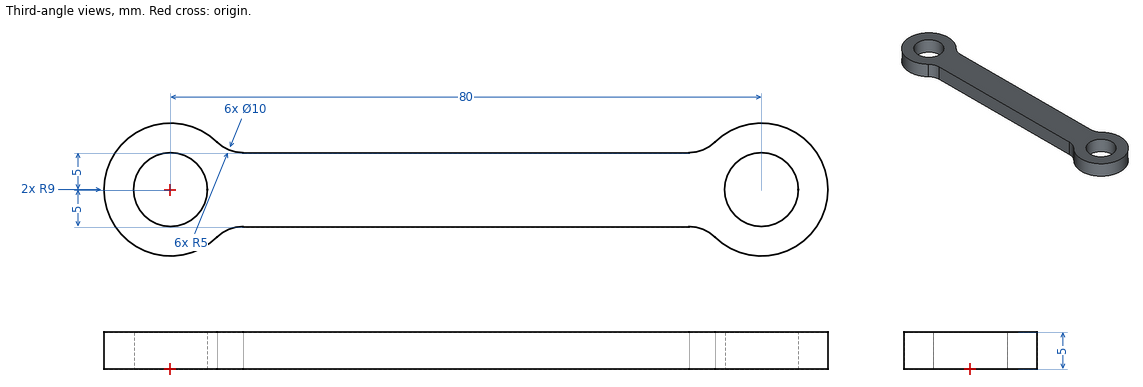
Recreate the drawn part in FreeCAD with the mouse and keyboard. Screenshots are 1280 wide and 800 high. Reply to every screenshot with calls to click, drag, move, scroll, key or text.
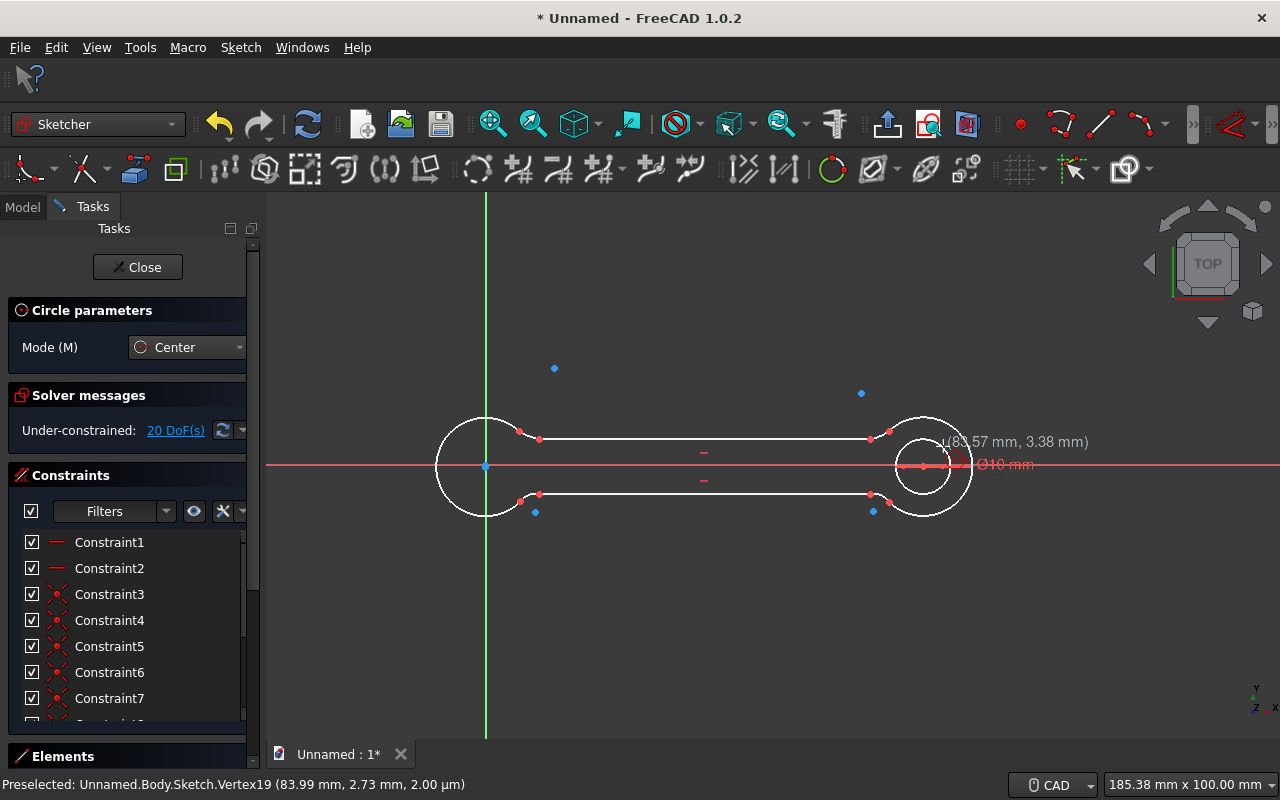
click(486, 465)
move(505, 446)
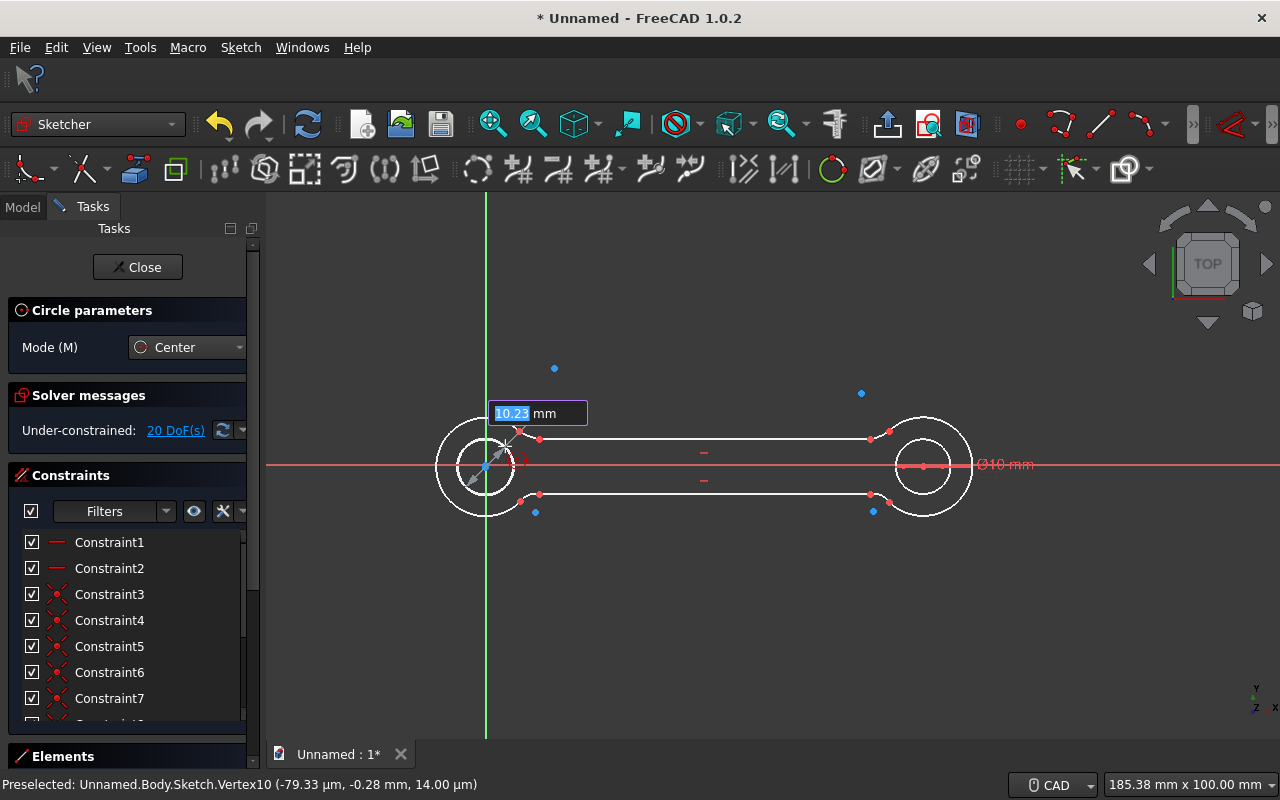
text(10)
key(Return)
key(Escape)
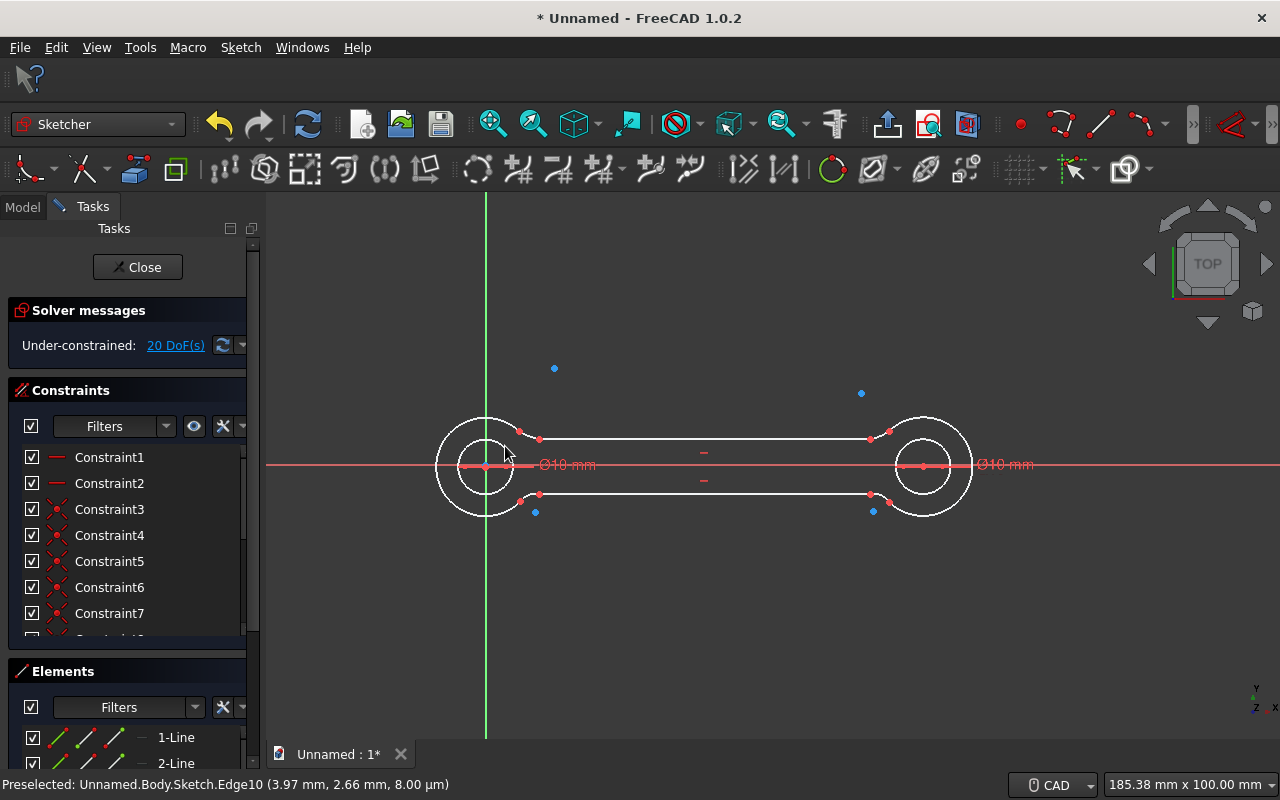
click(771, 439)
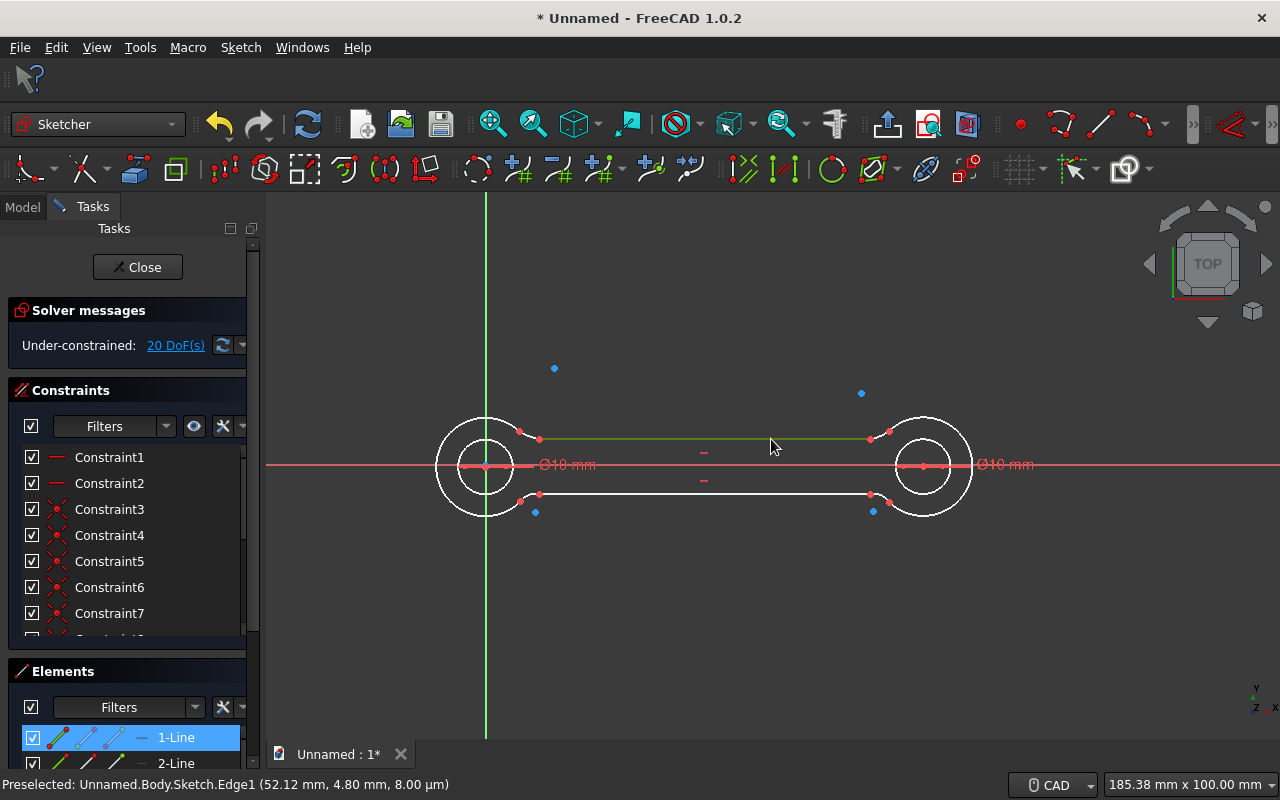
scroll(529, 436, up, 2)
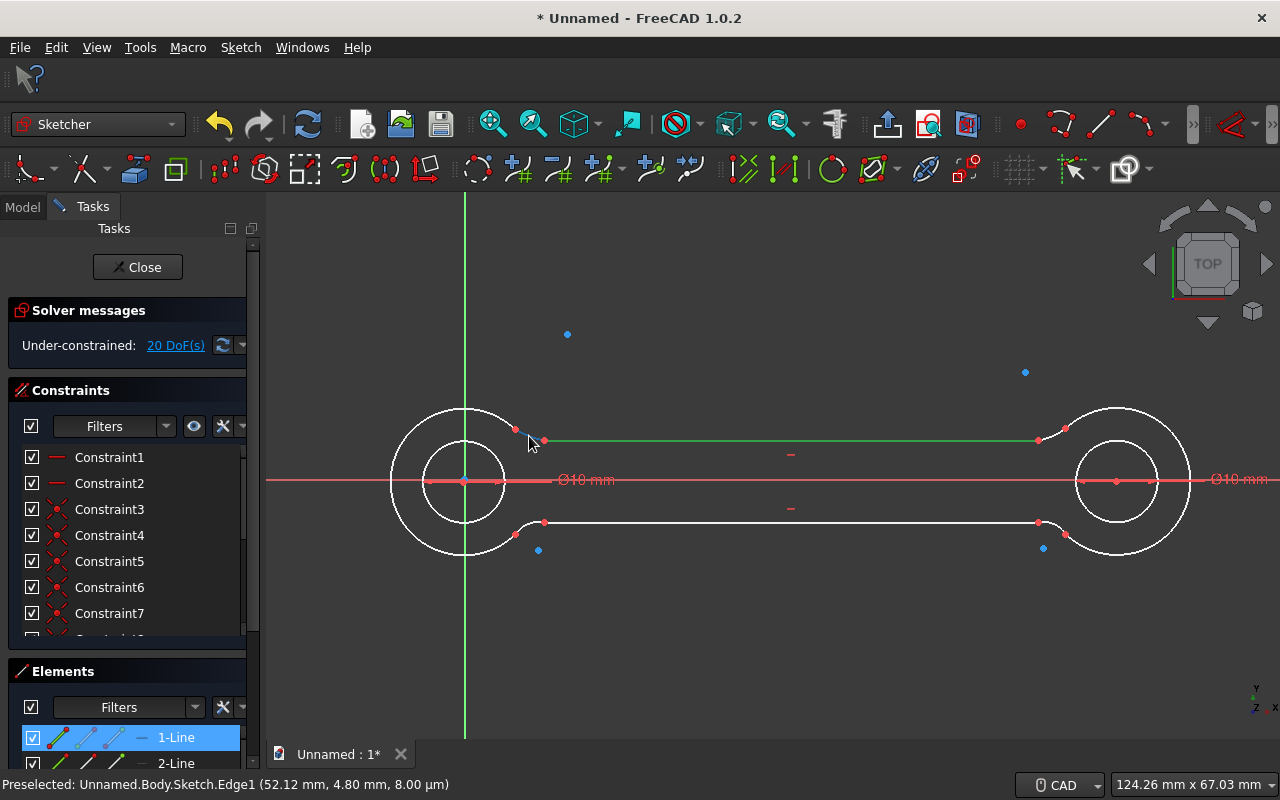
click(529, 436)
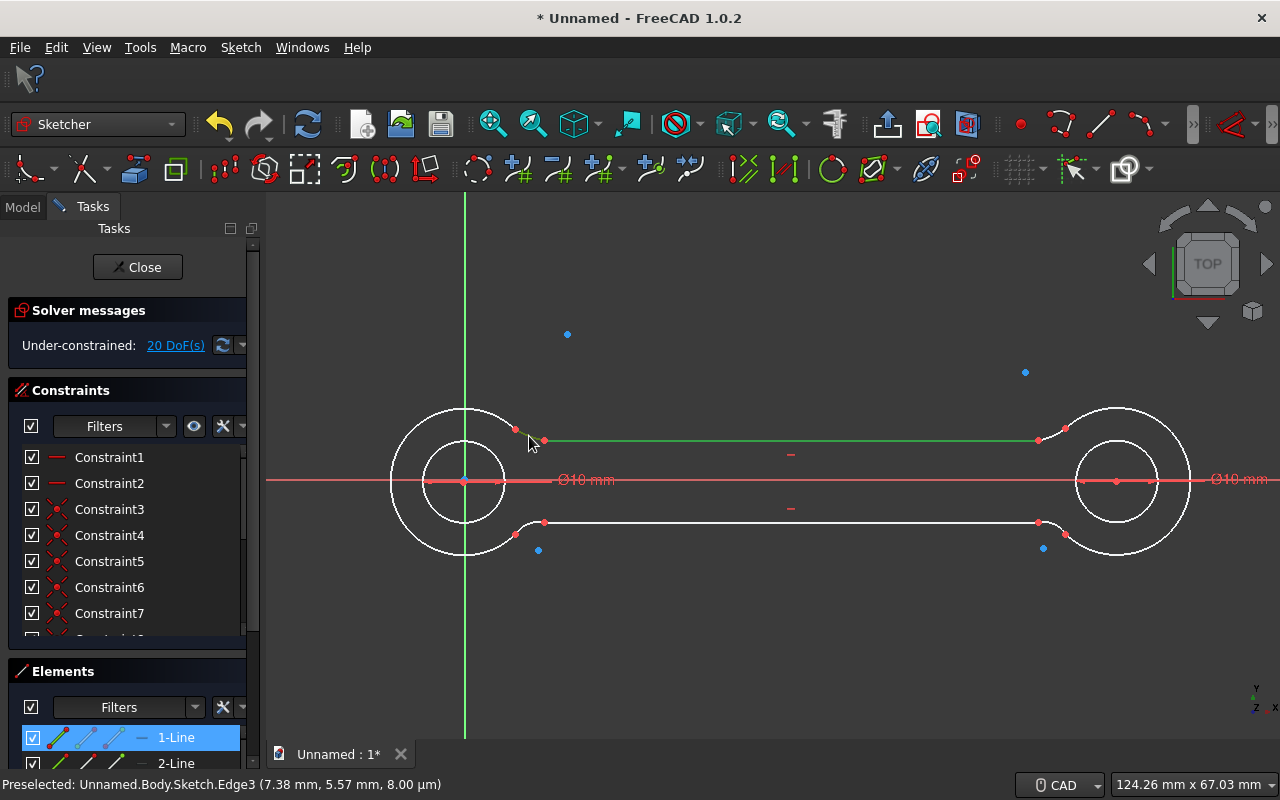
key(t)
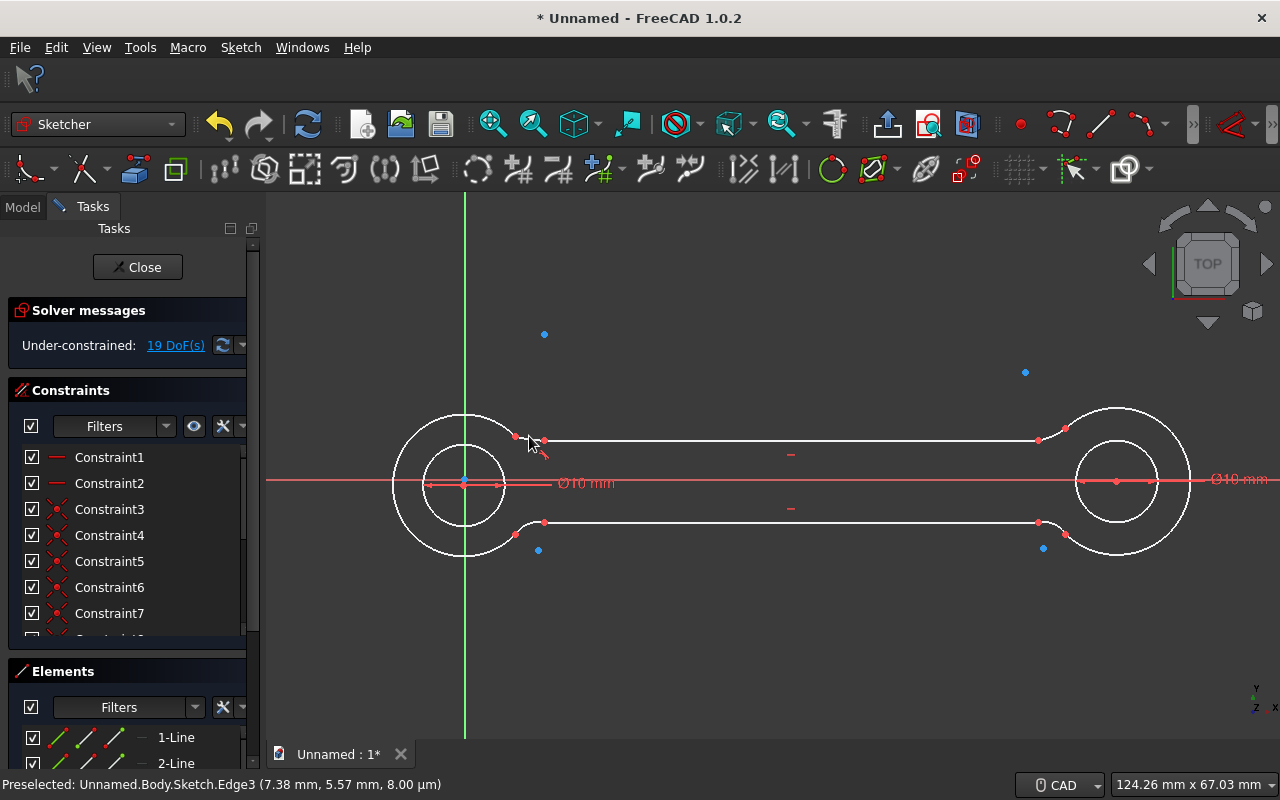
click(890, 441)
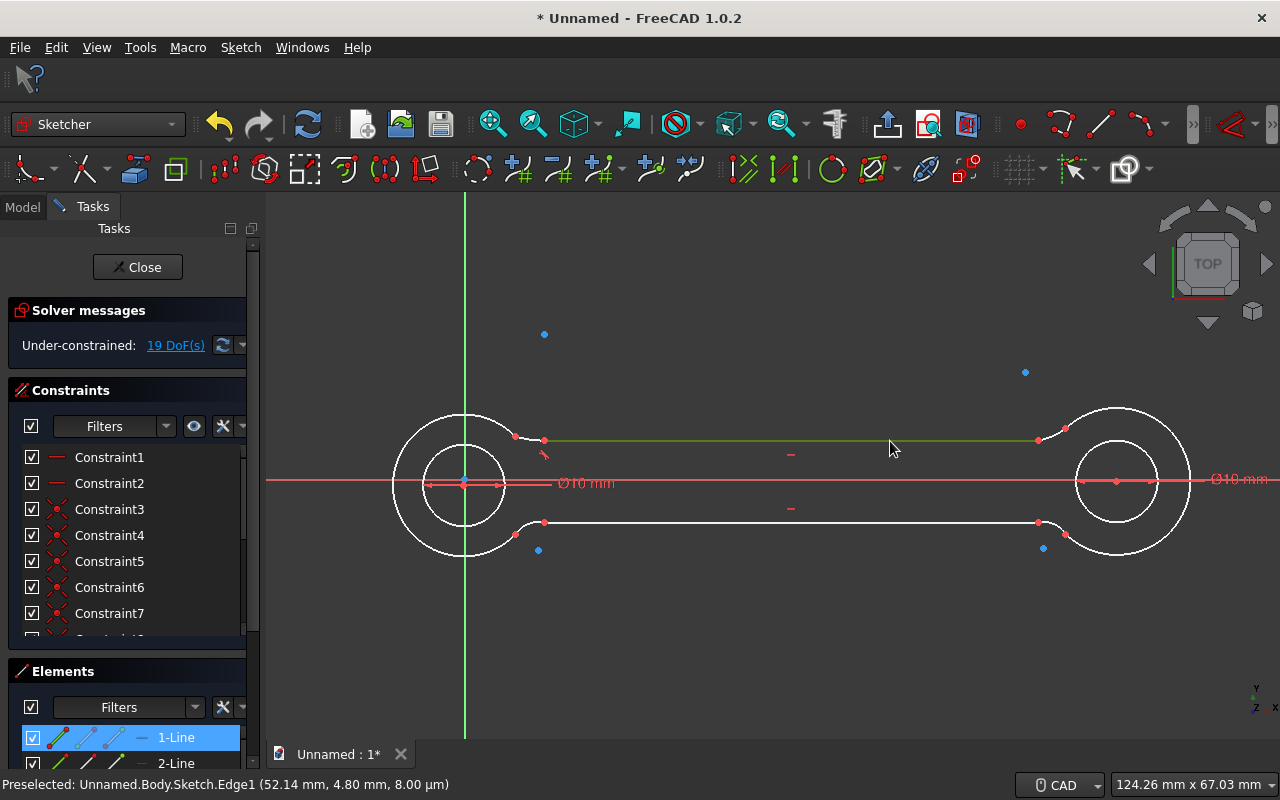
scroll(1047, 438, up, 3)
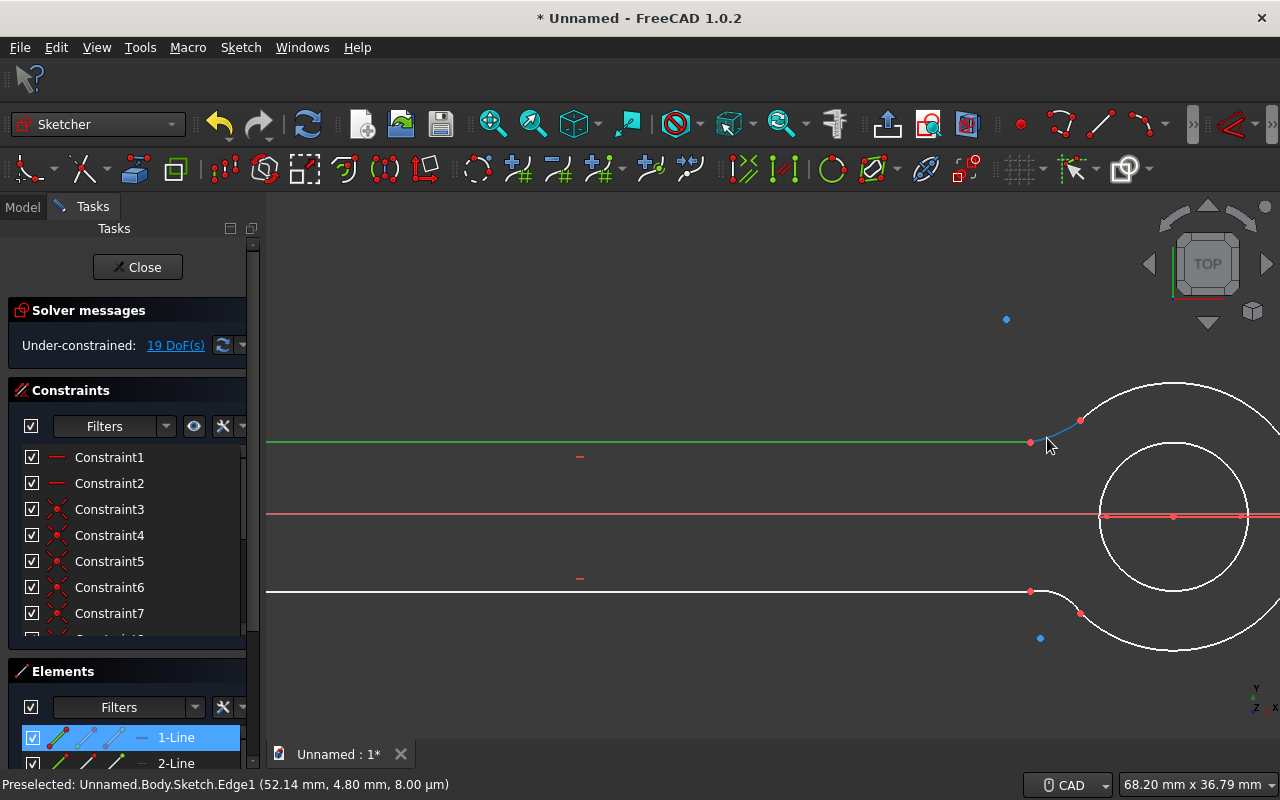
click(1046, 438)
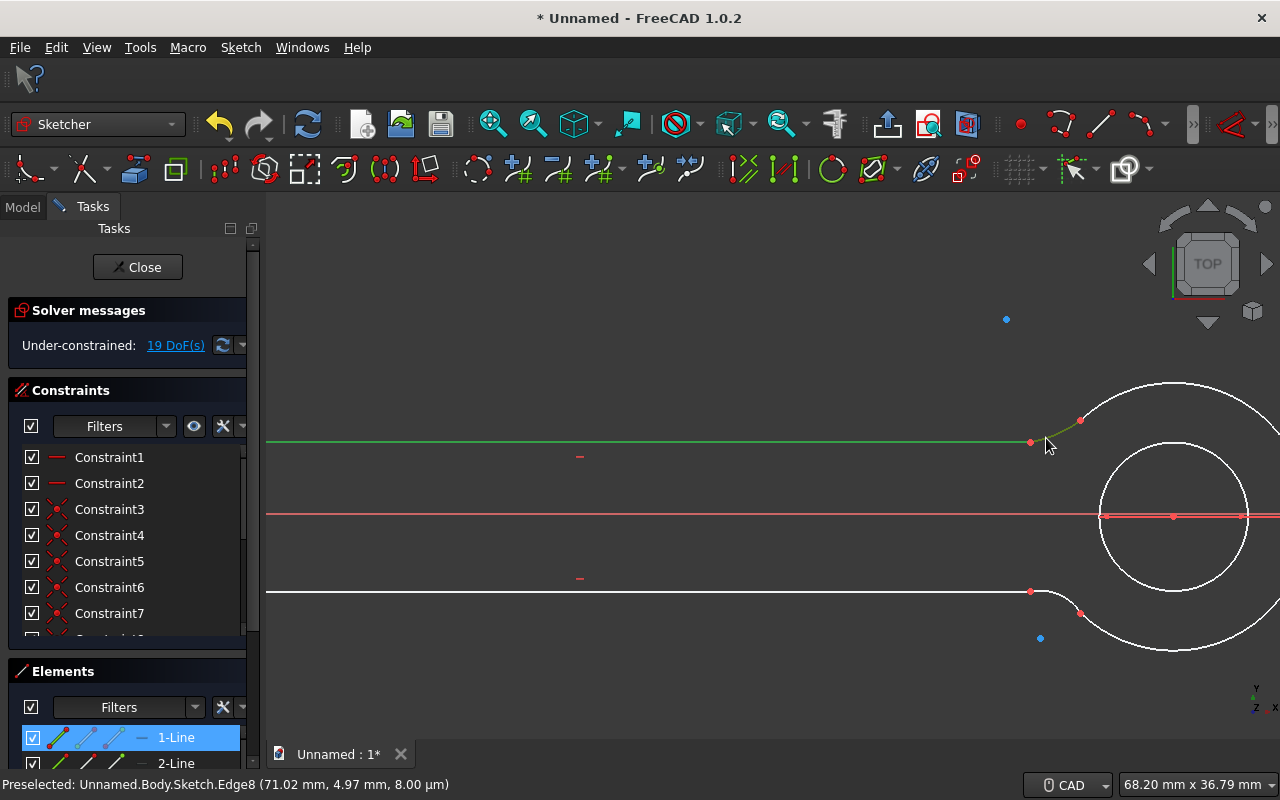
key(t)